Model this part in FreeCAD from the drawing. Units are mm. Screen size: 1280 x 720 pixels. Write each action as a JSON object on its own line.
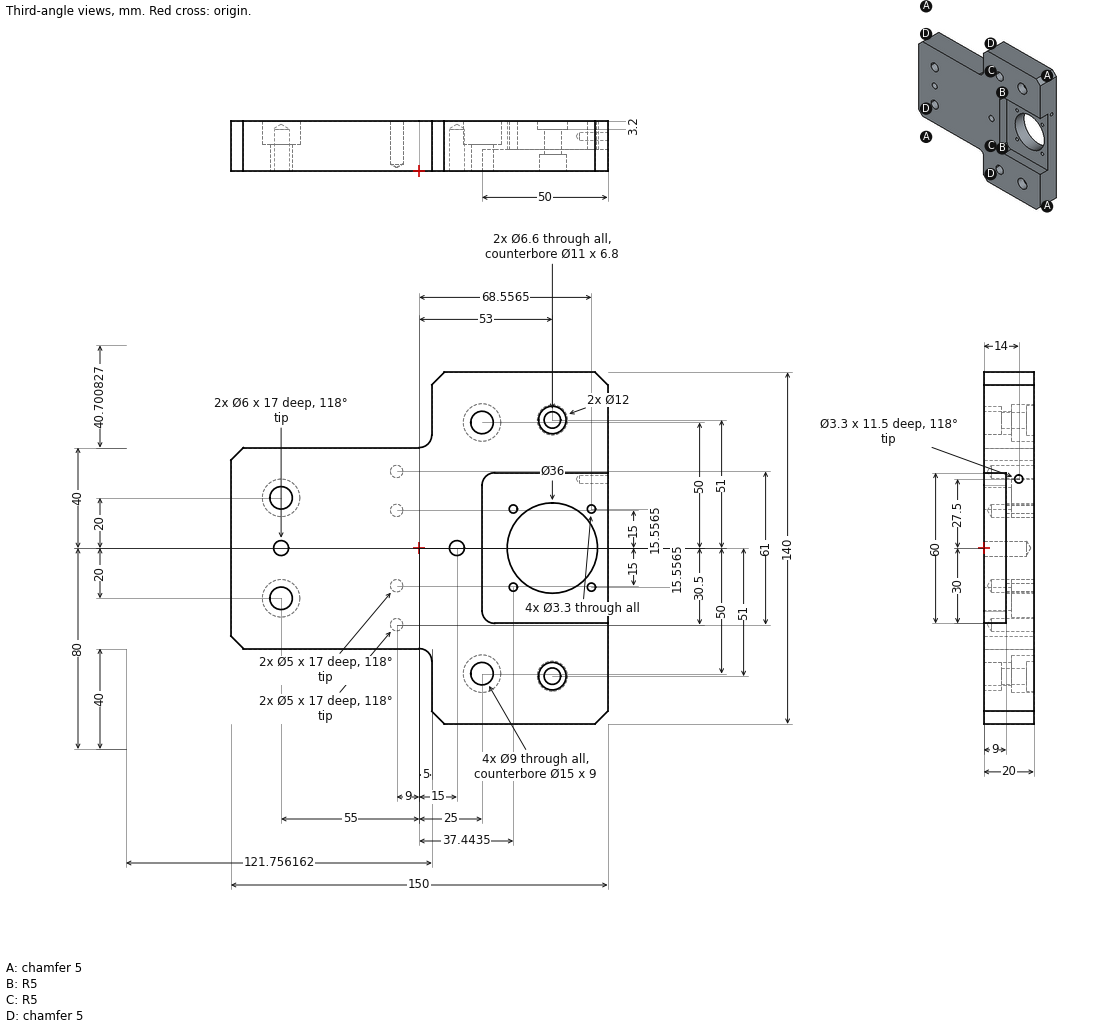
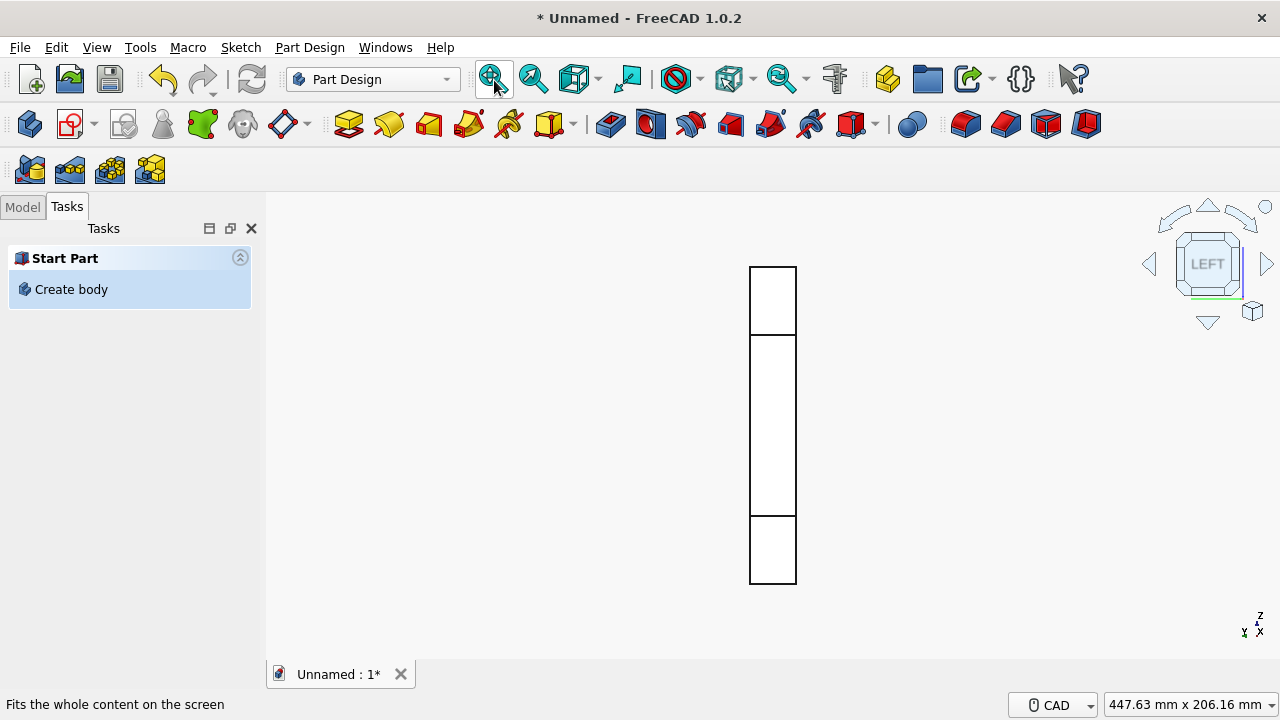
{"action": "key", "text": "v 3"}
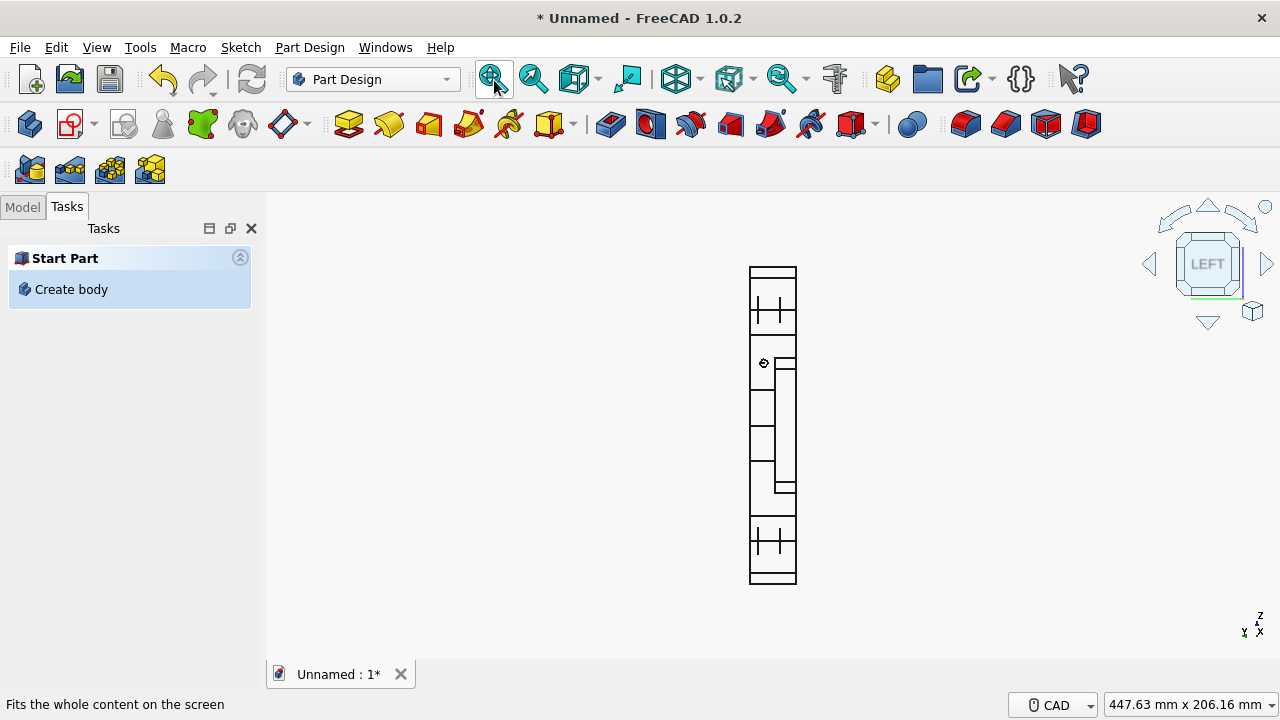
{"action": "key", "text": "0"}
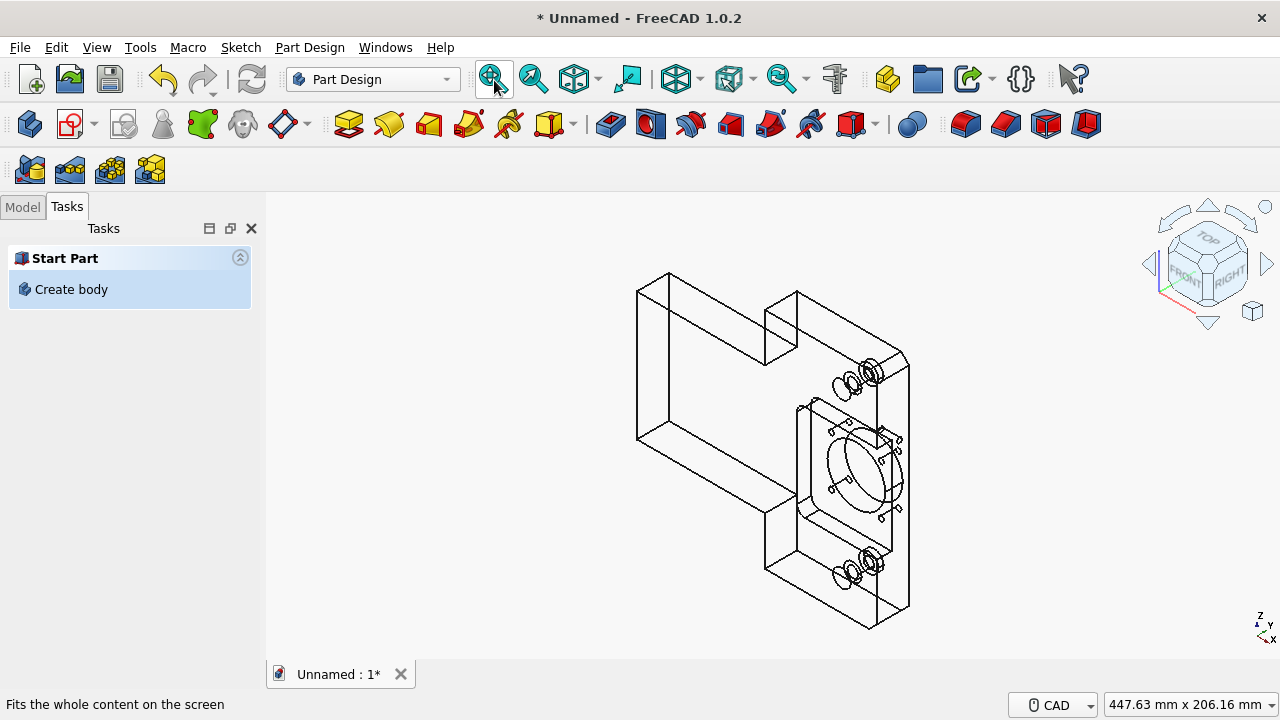
{"action": "left_click", "coordinate": [781, 503]}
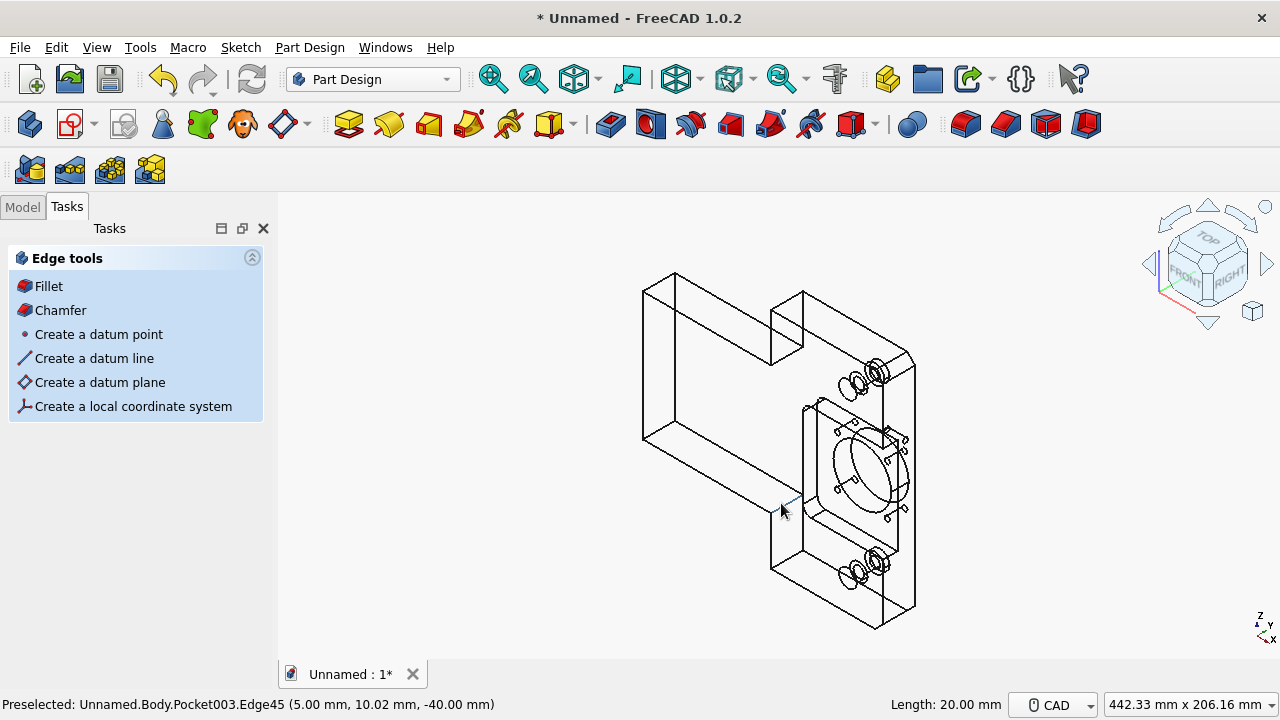
{"action": "left_click", "coordinate": [787, 355], "text": "ctrl"}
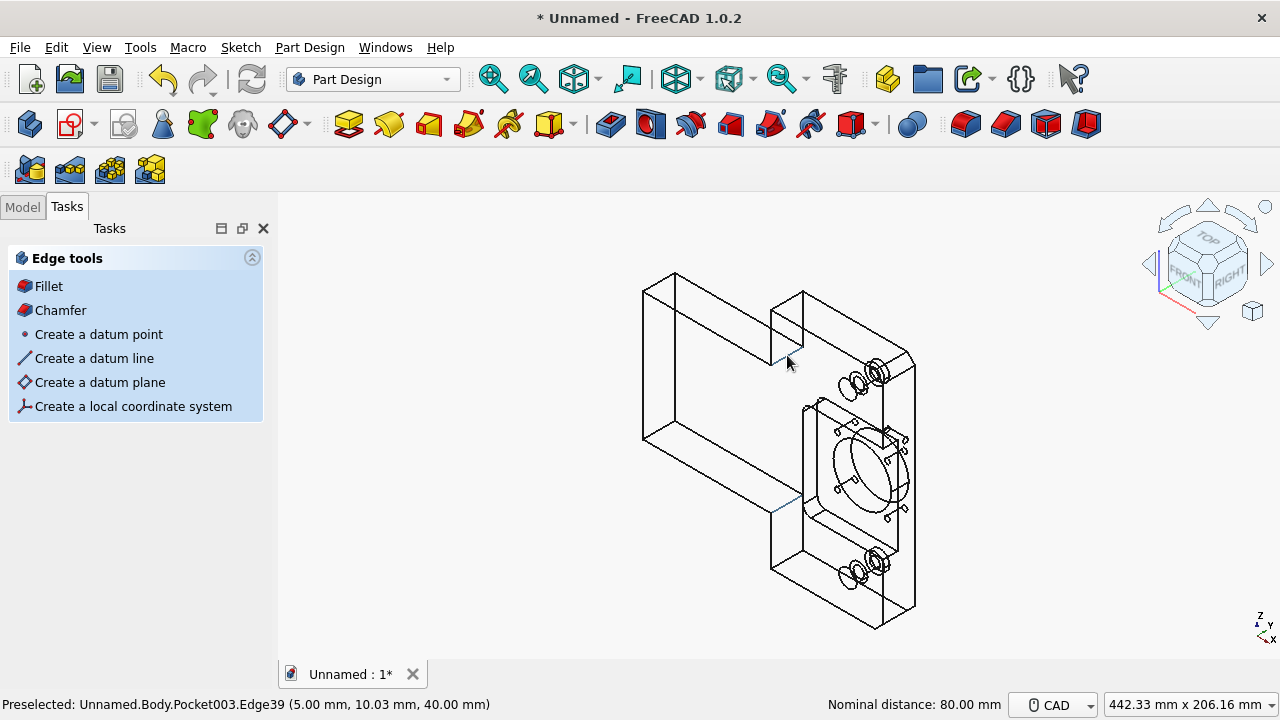
{"action": "key", "text": "v 1"}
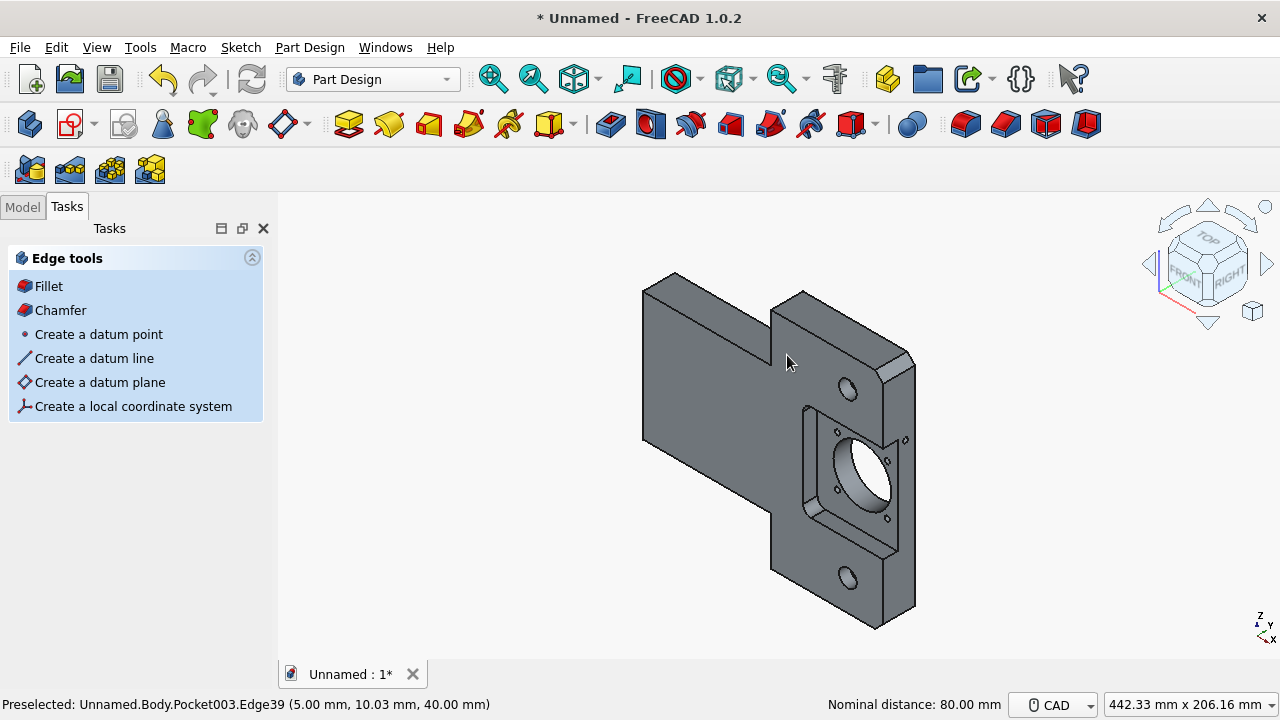
{"action": "left_click", "coordinate": [966, 124]}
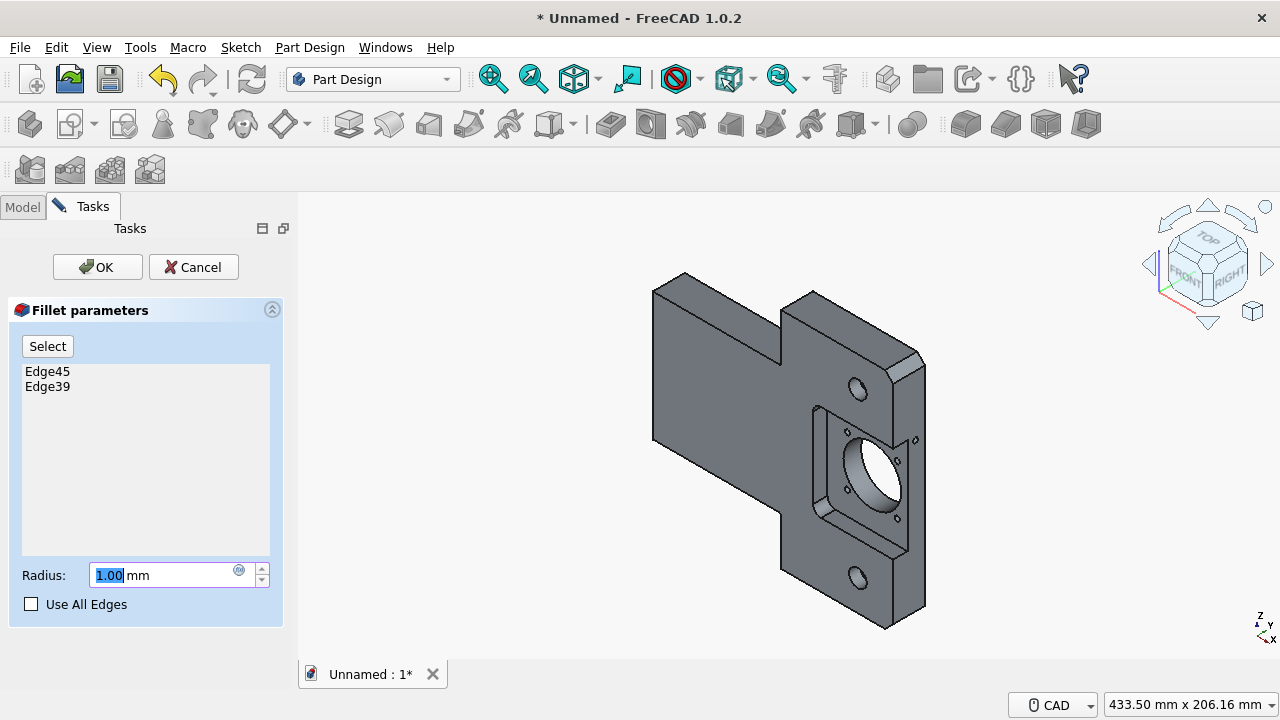
{"action": "type", "text": "5"}
{"action": "key", "text": "Tab"}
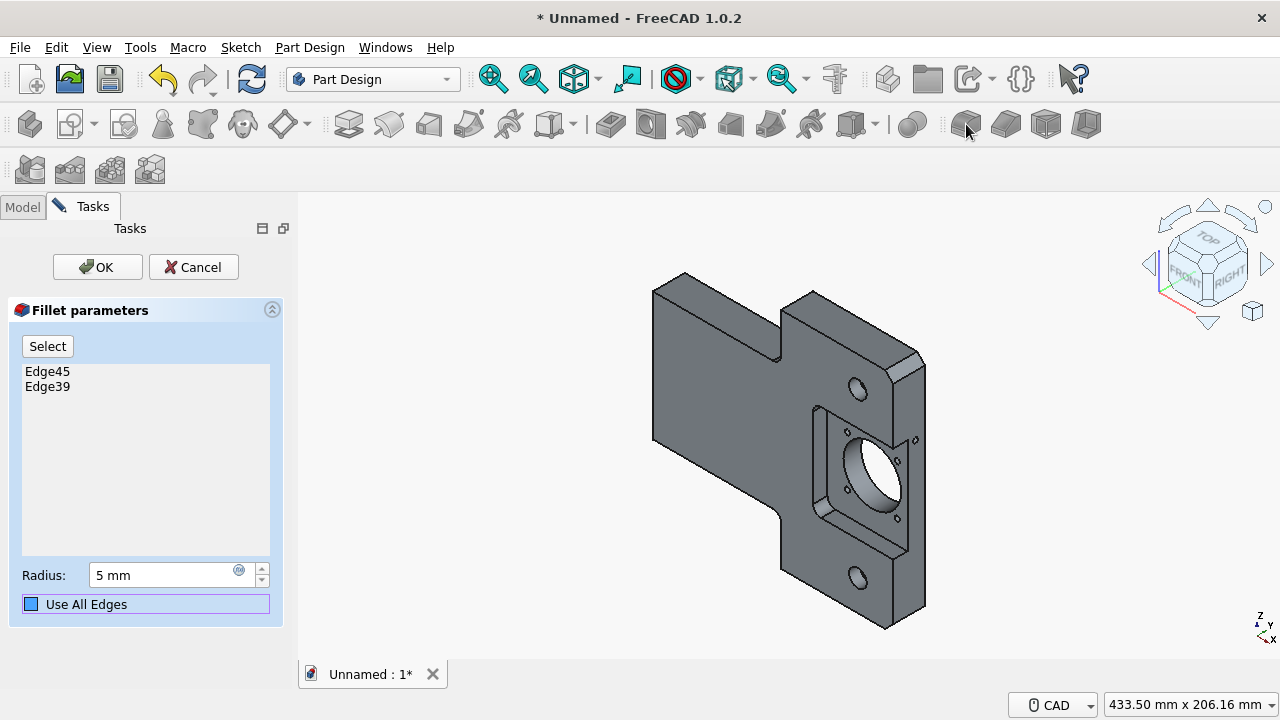
{"action": "left_click", "coordinate": [98, 267]}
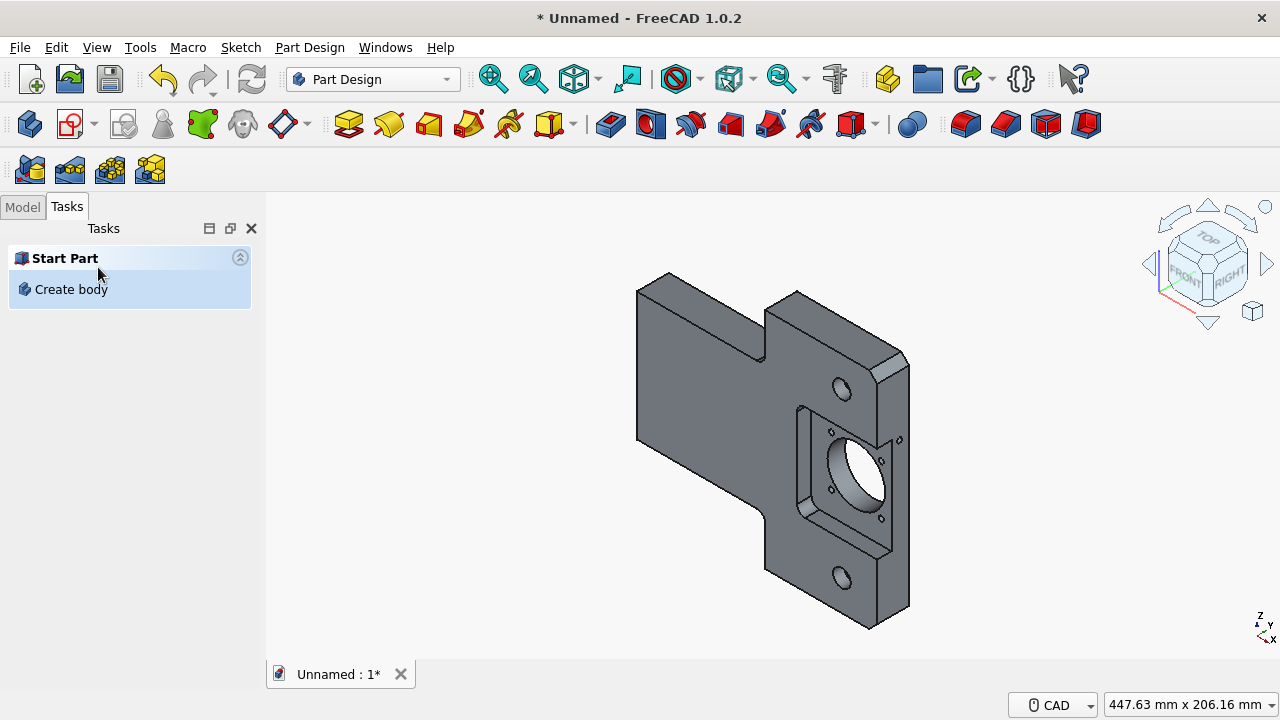
{"action": "key", "text": "2"}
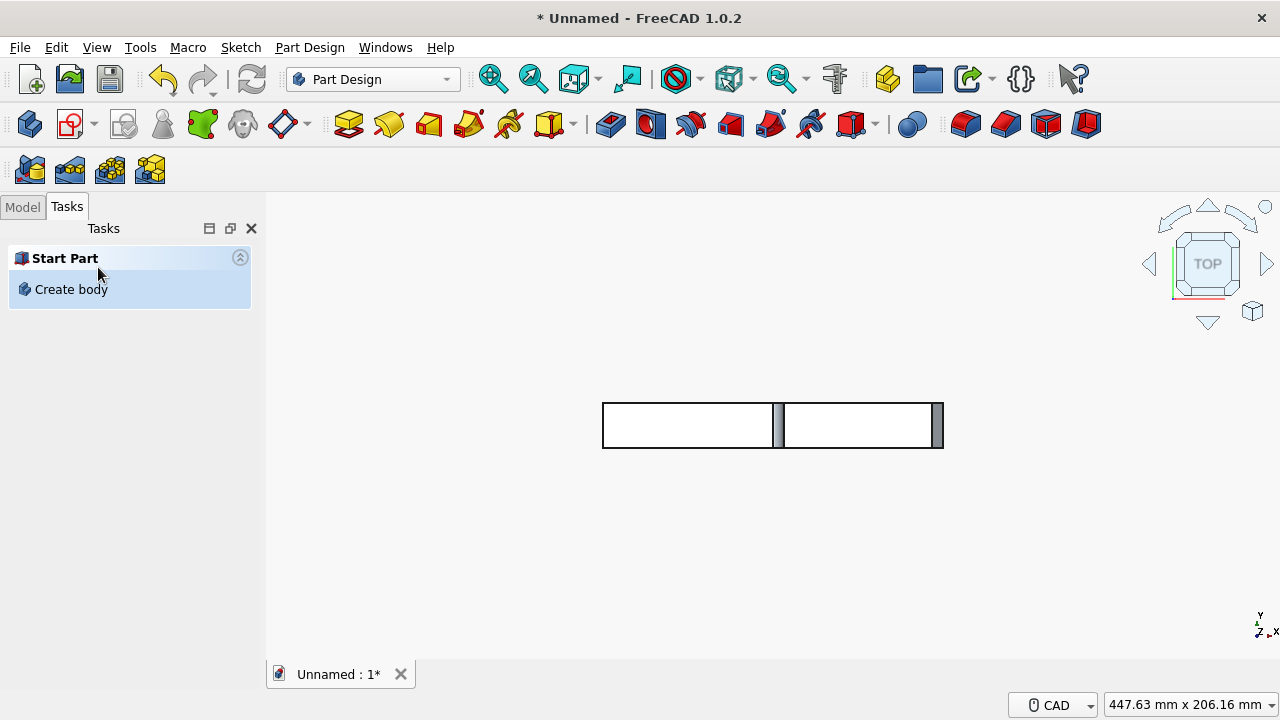
{"action": "left_click", "coordinate": [494, 80]}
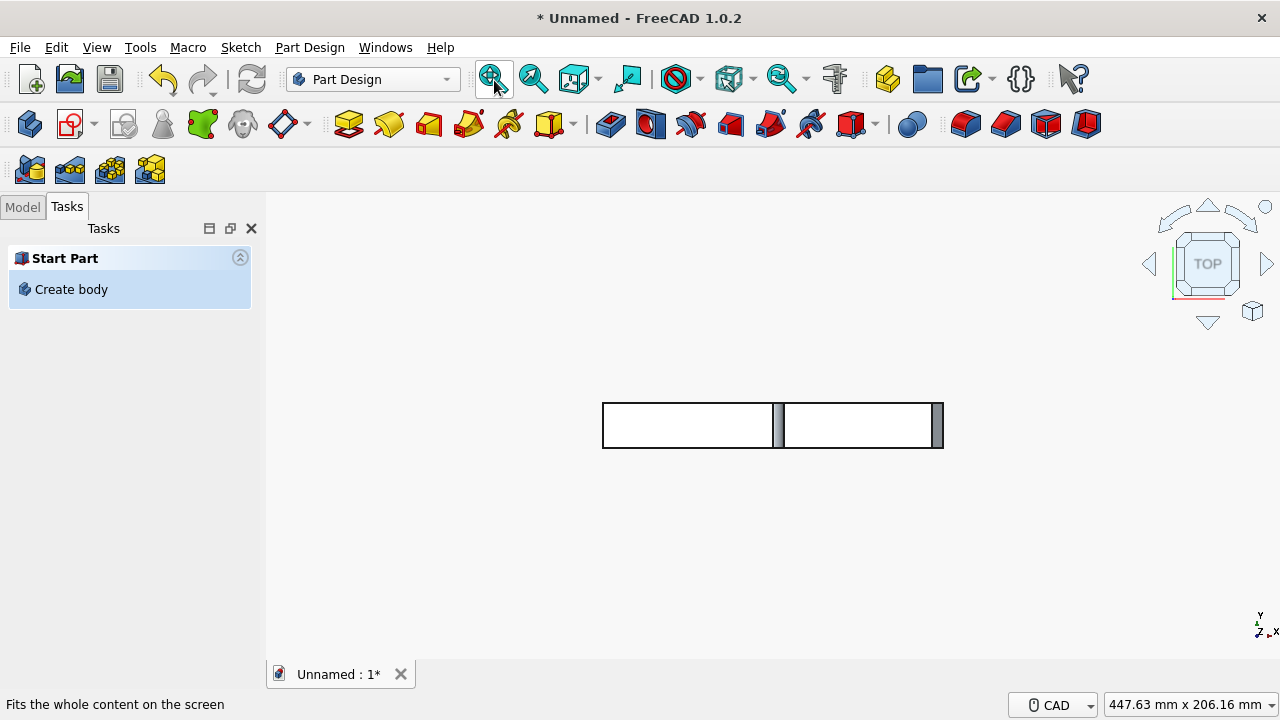
{"action": "left_click", "coordinate": [784, 424]}